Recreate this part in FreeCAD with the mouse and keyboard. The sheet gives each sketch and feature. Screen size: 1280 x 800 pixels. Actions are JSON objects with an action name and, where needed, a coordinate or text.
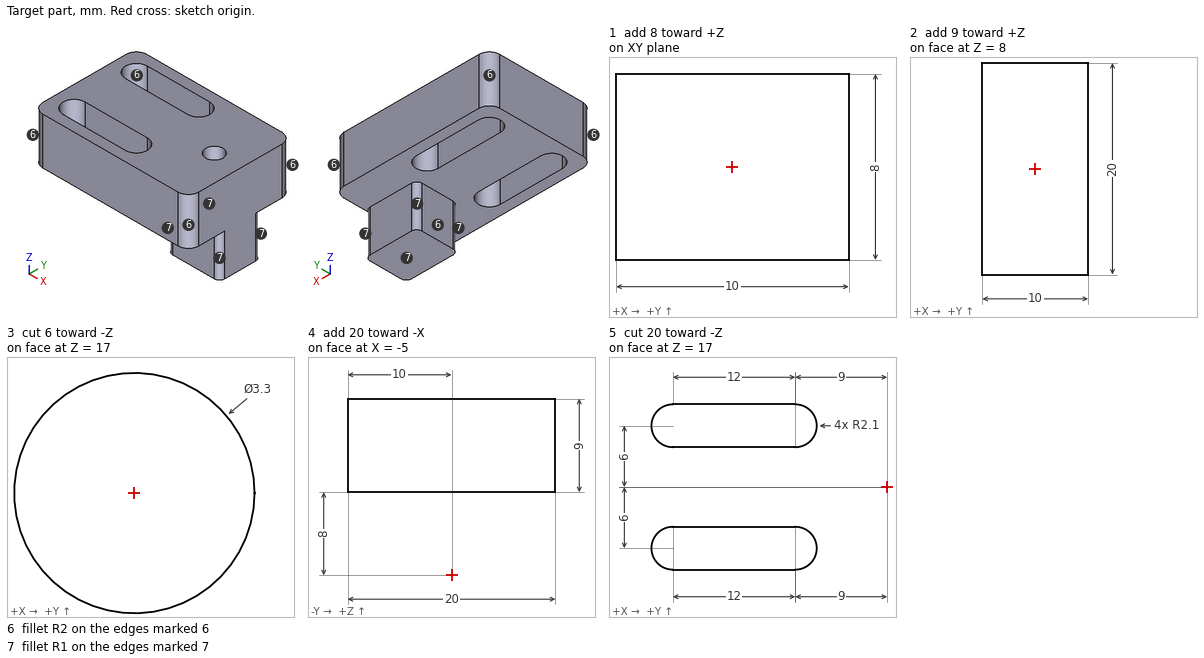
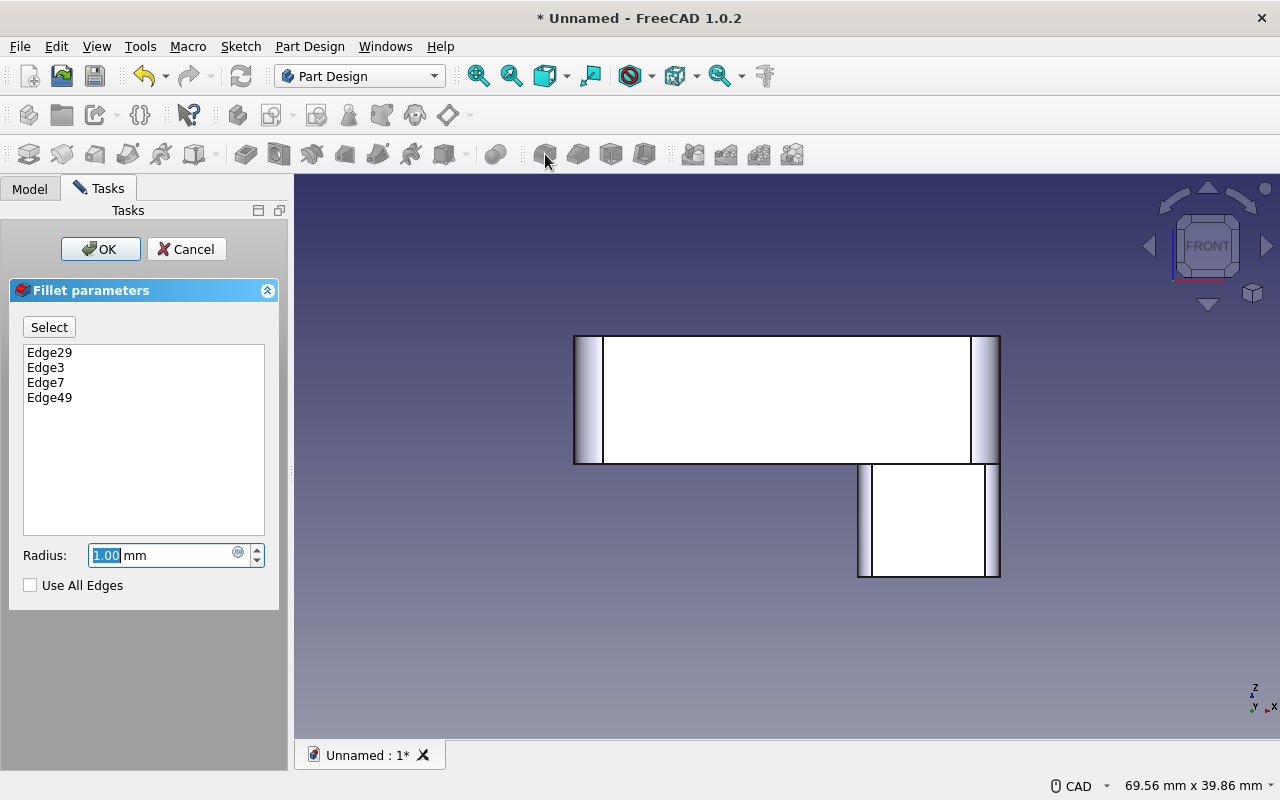
{"action": "type", "text": "1"}
{"action": "key", "text": "Tab"}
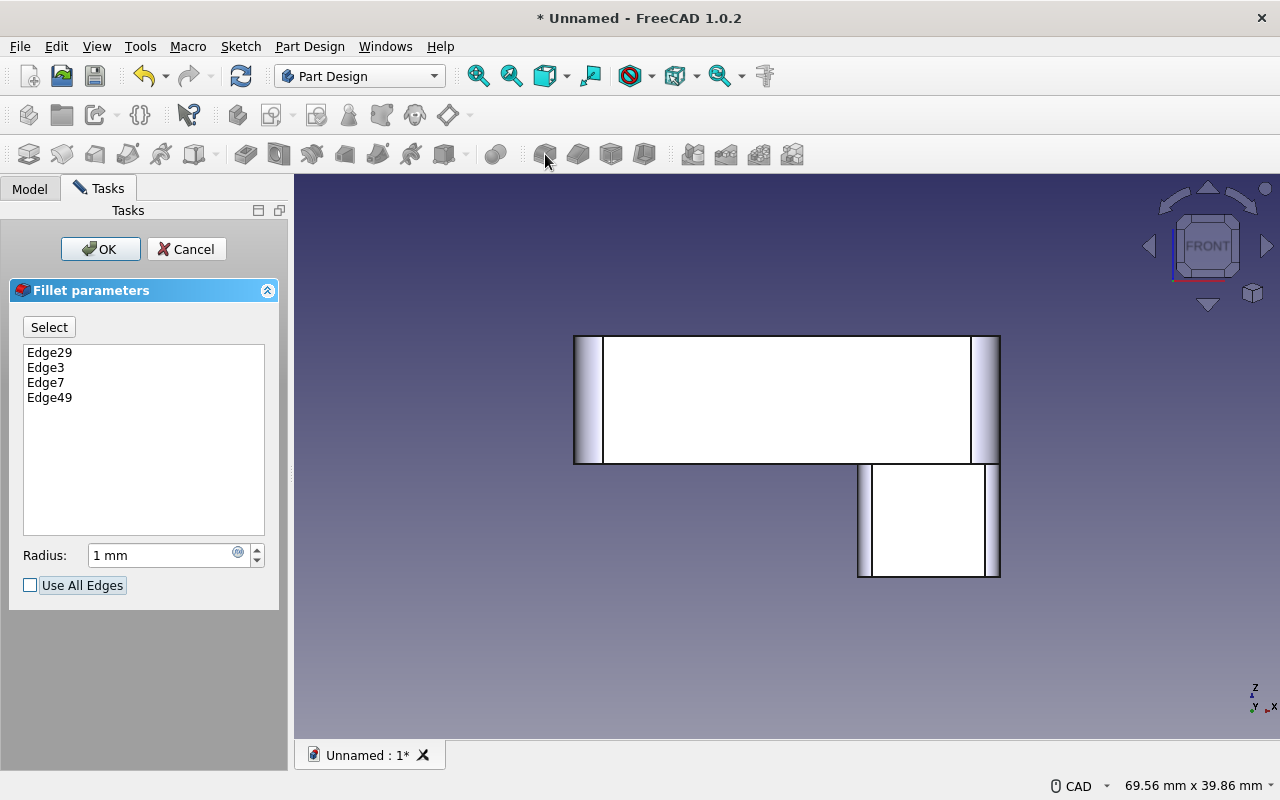
{"action": "left_click", "coordinate": [101, 249]}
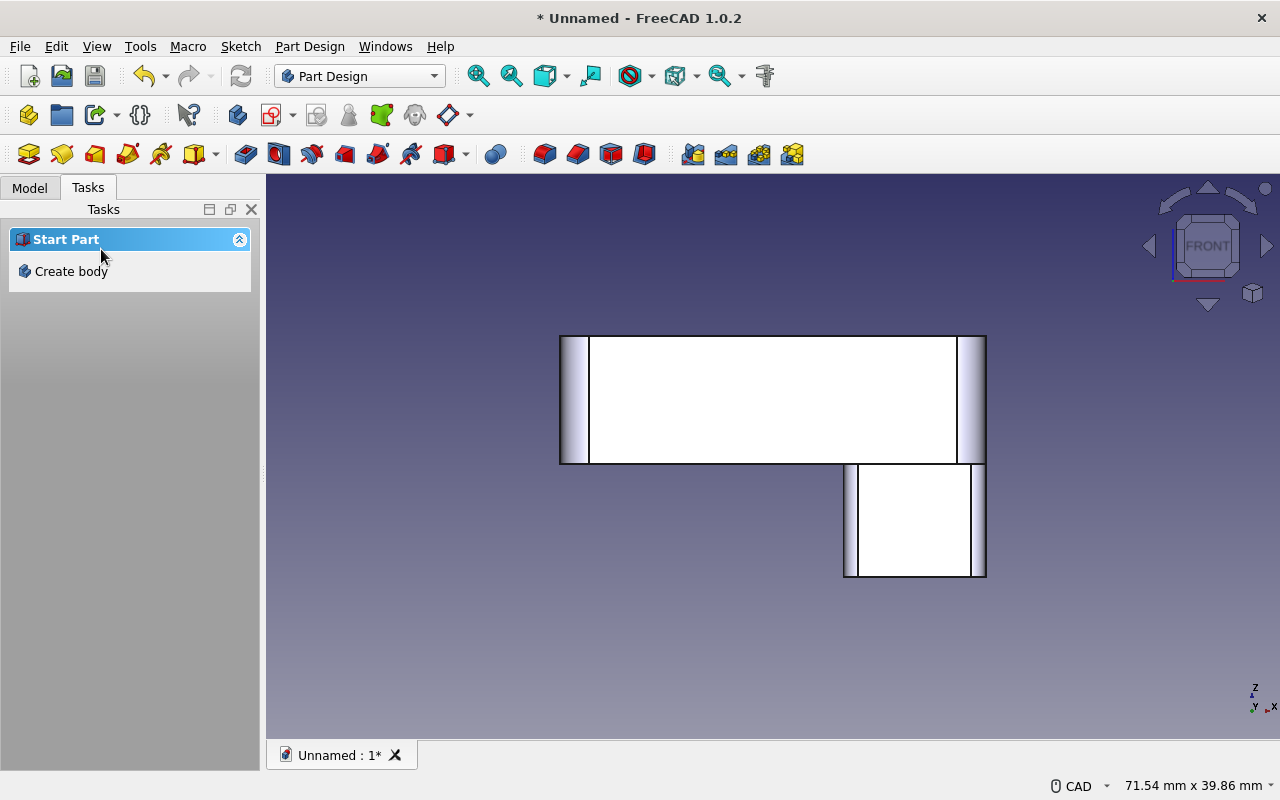
{"action": "key", "text": "0"}